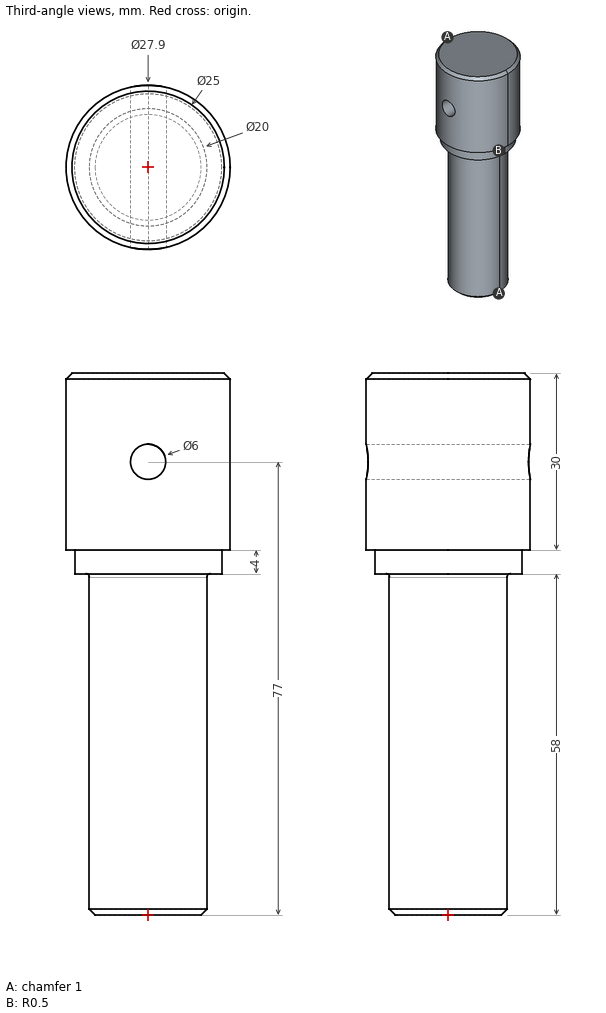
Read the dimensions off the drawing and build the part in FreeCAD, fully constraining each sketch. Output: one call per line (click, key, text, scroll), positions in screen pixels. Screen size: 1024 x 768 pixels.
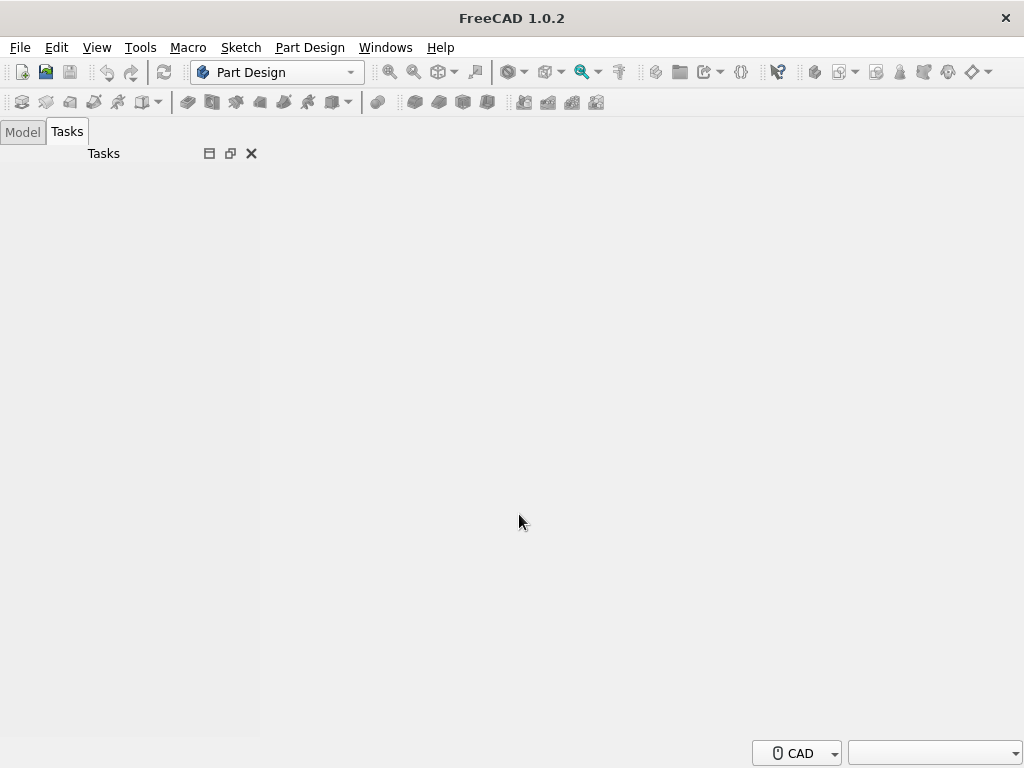
click(22, 72)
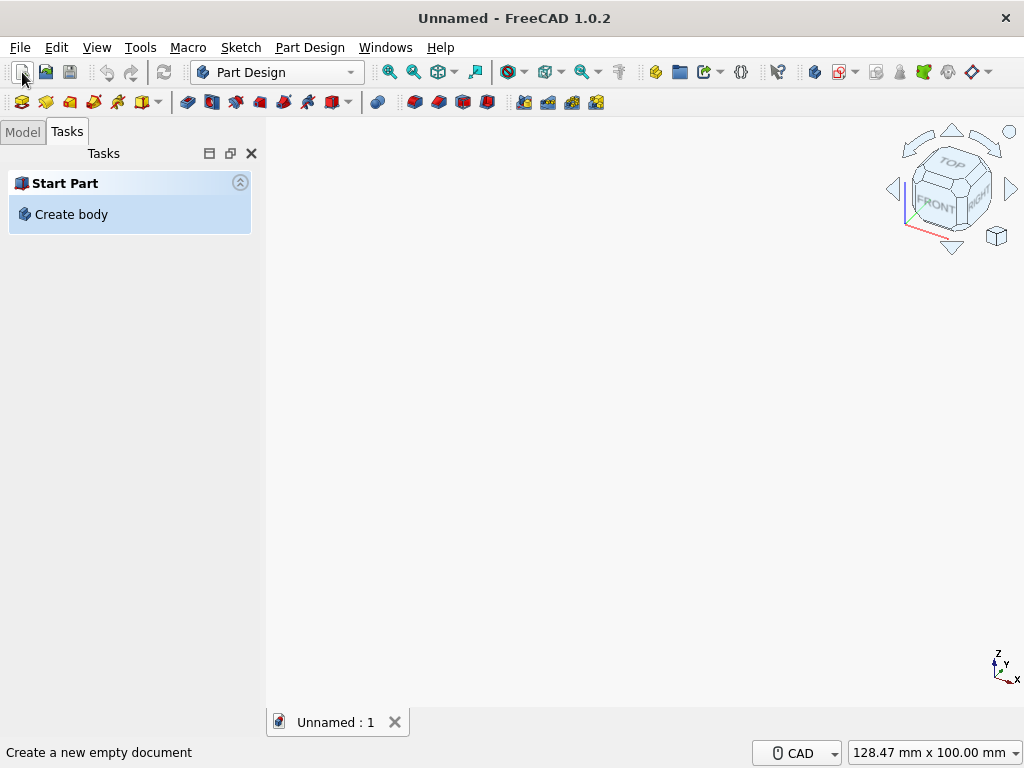
click(840, 72)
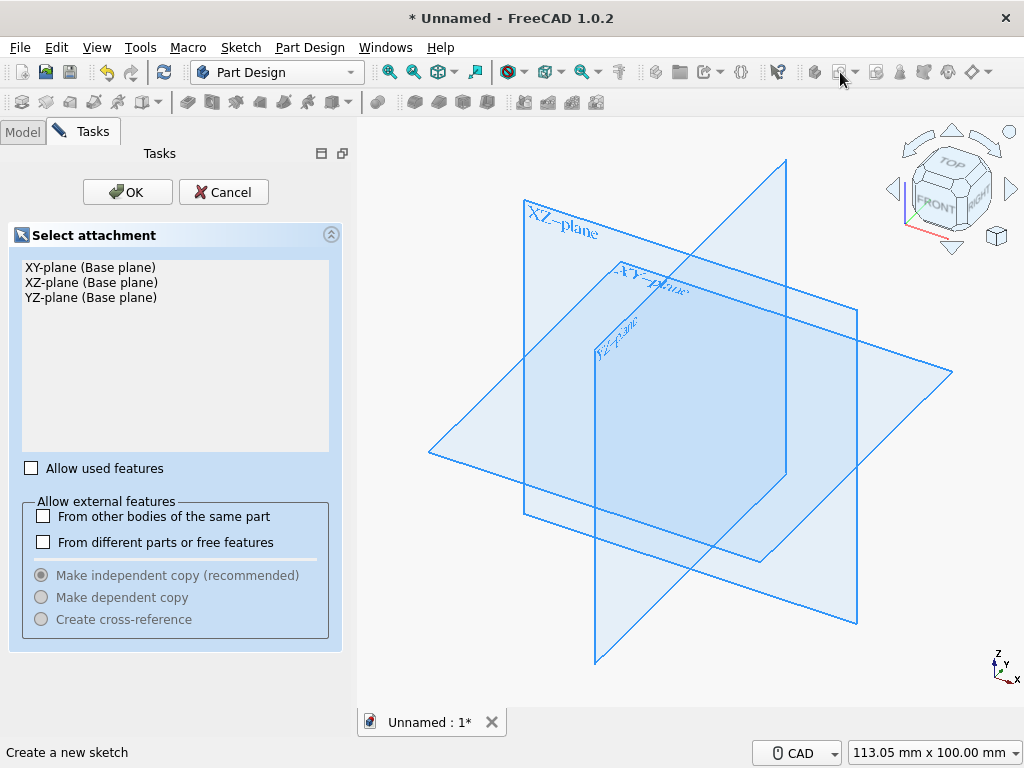
click(82, 268)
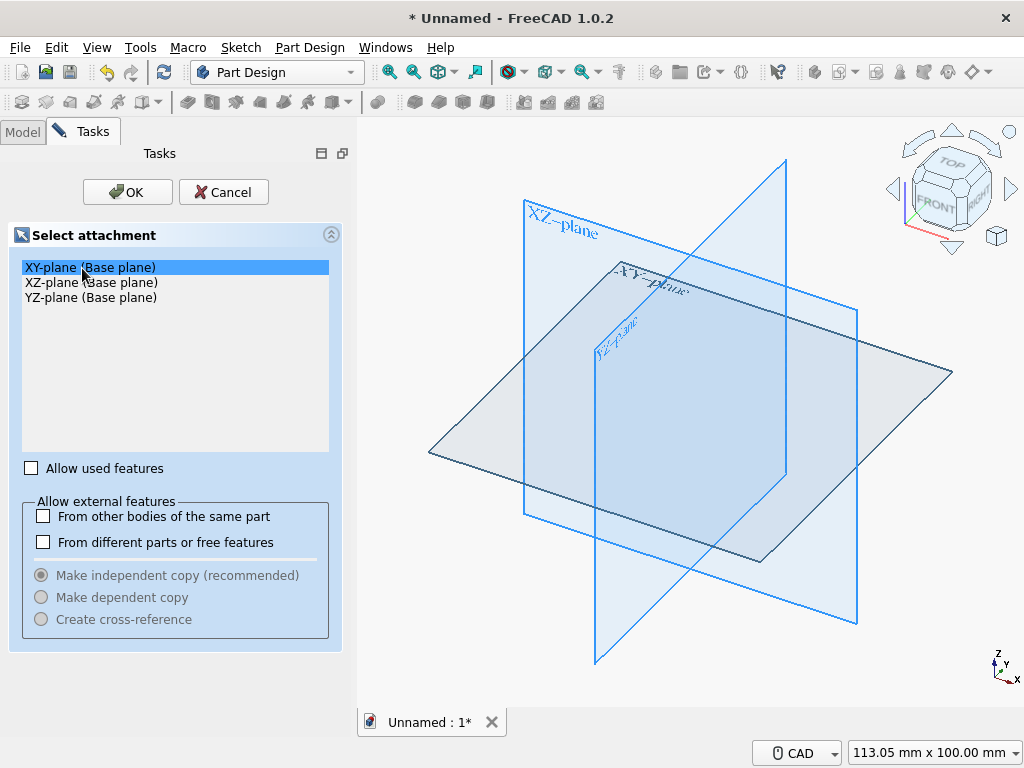
click(128, 192)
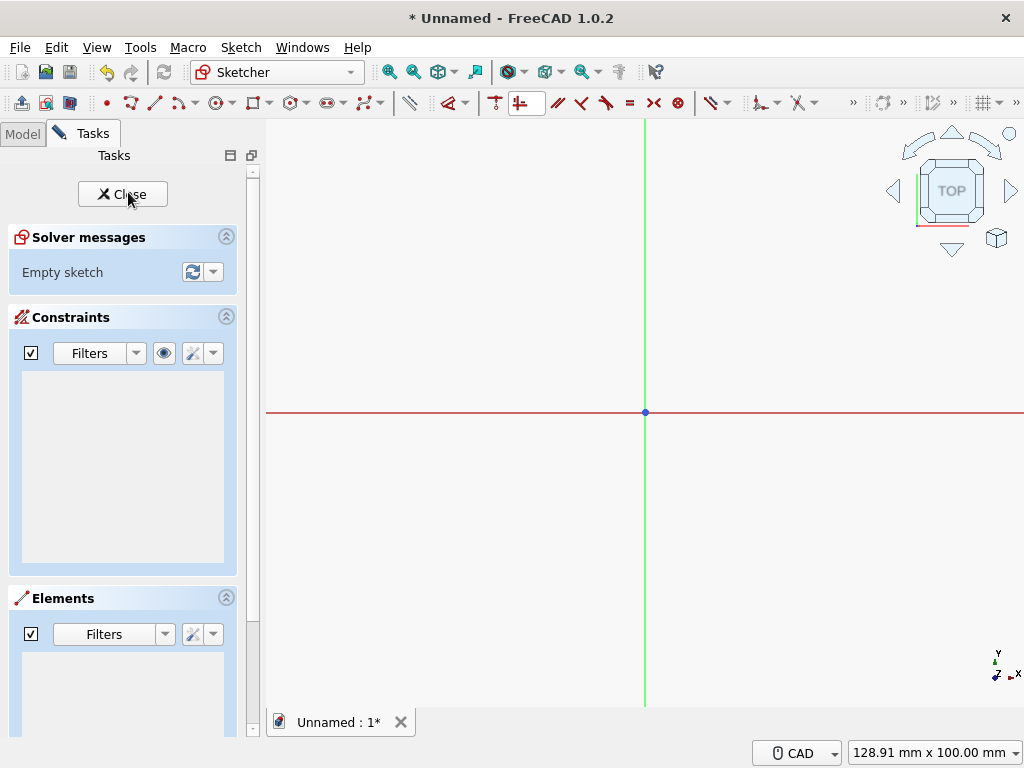
scroll(675, 413, up, 6)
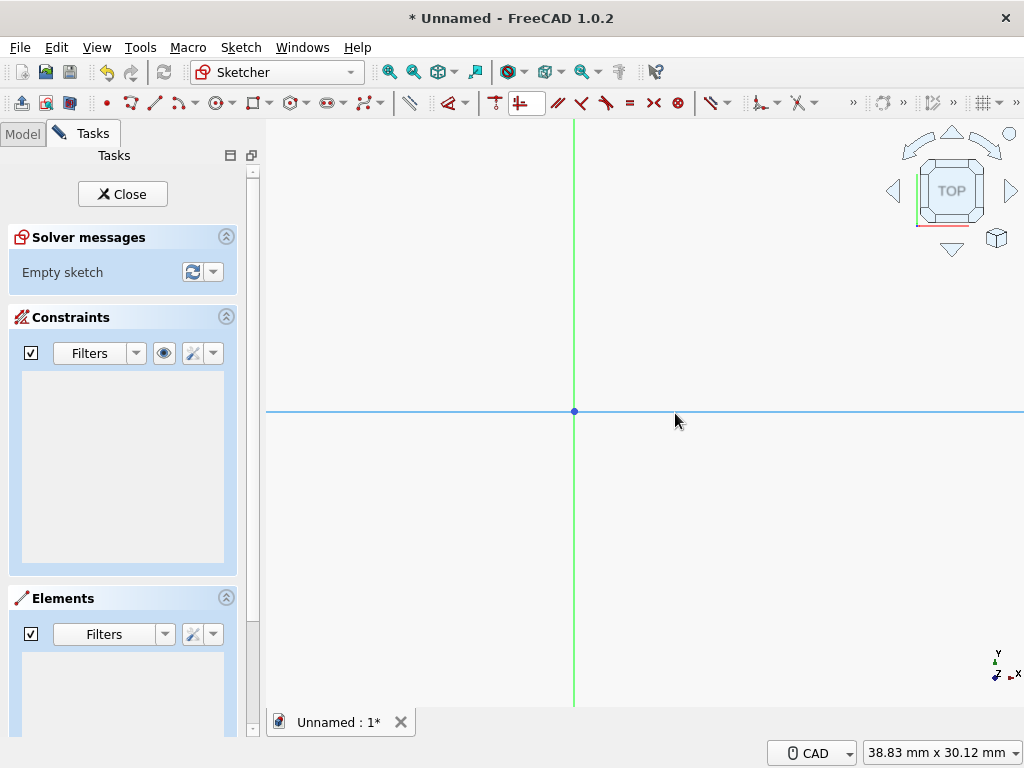
click(216, 104)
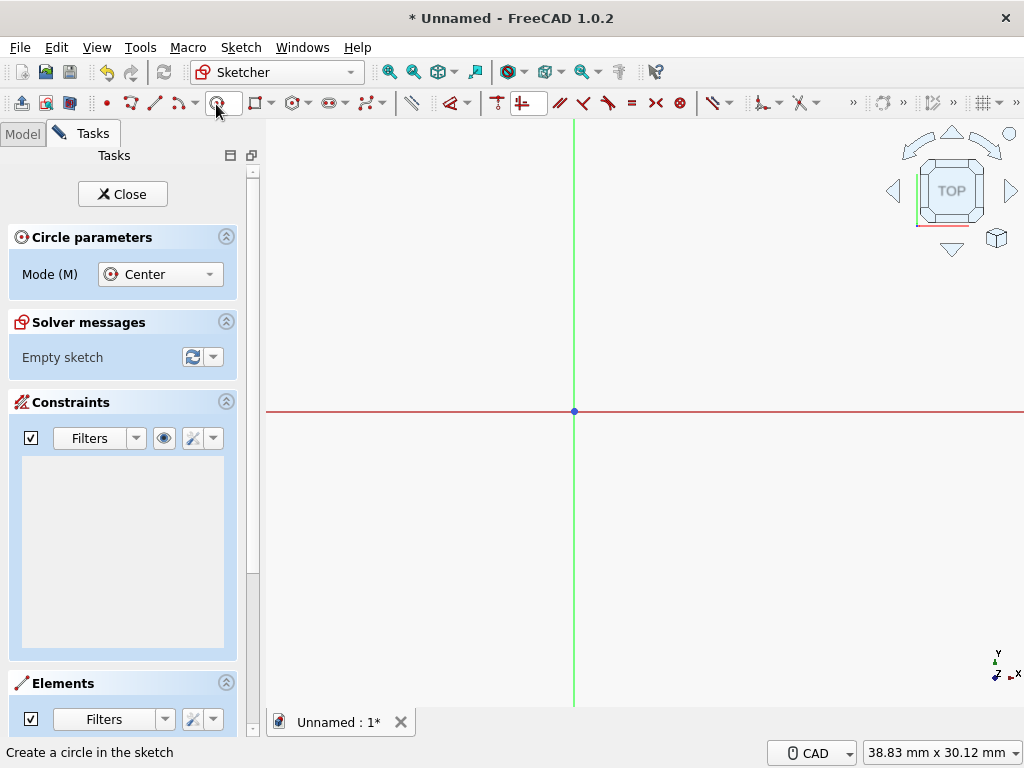
click(574, 412)
click(712, 274)
key(Escape)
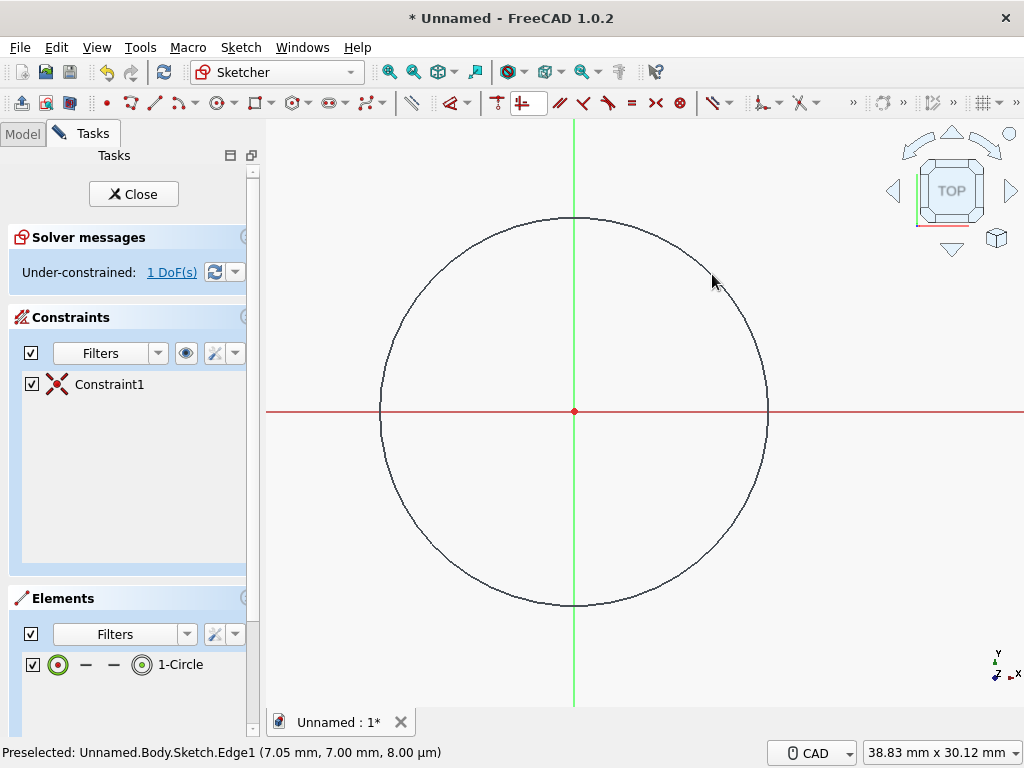
click(450, 104)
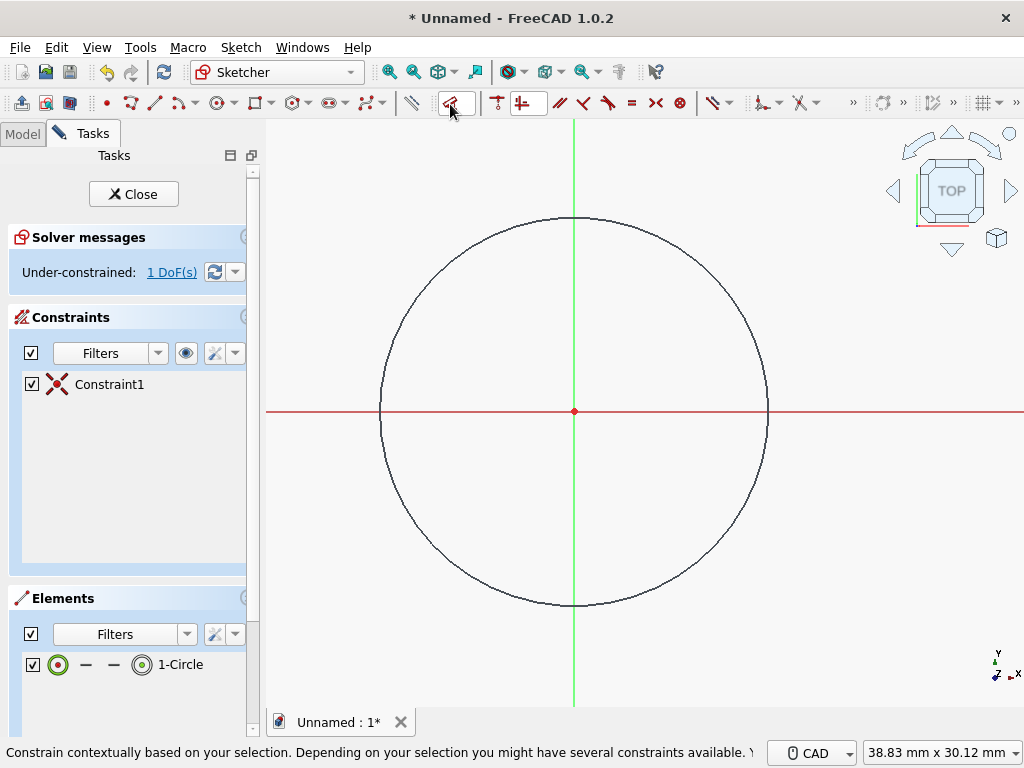
click(711, 274)
click(734, 251)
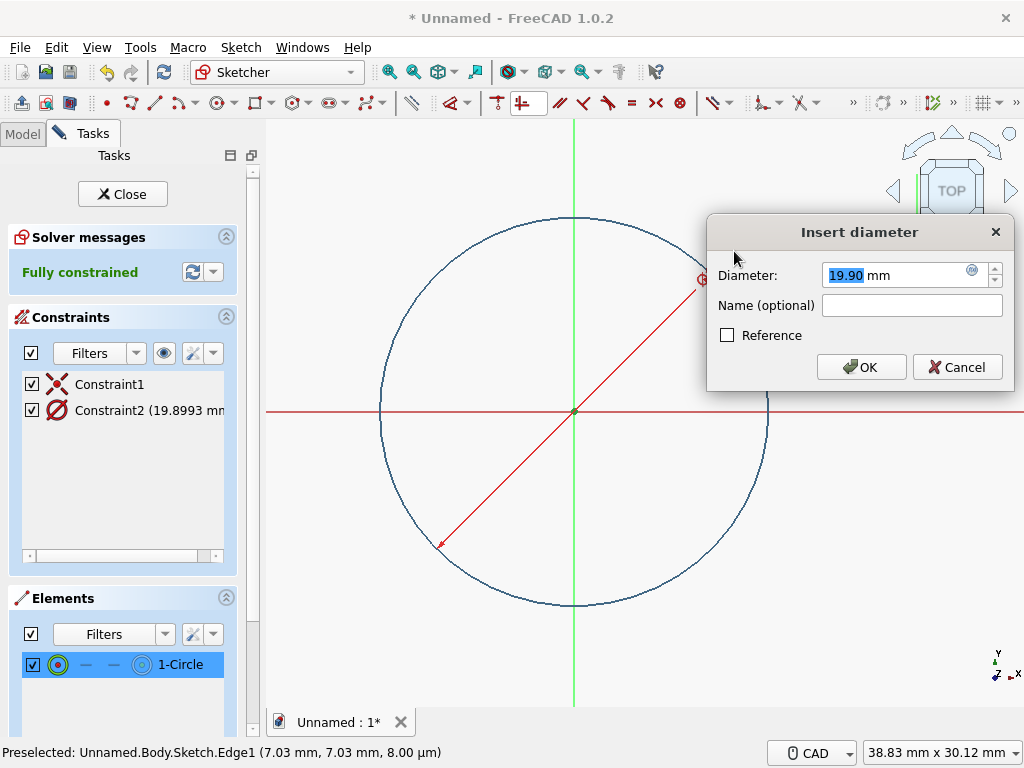
text(20)
key(Return)
key(Escape)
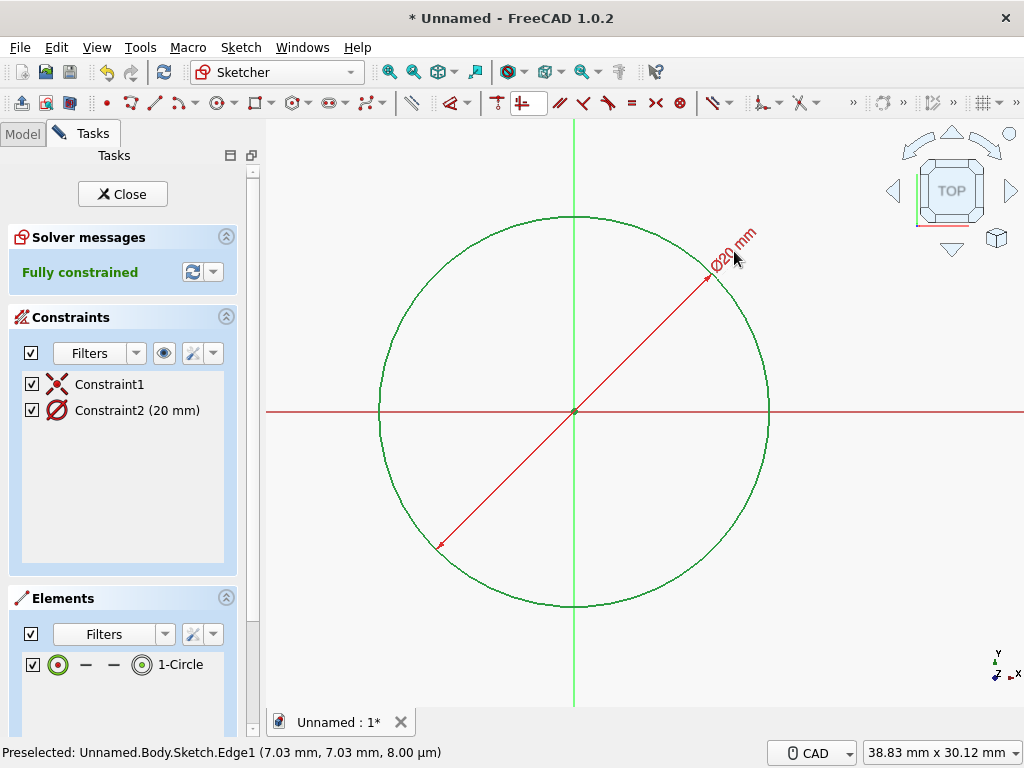
click(123, 194)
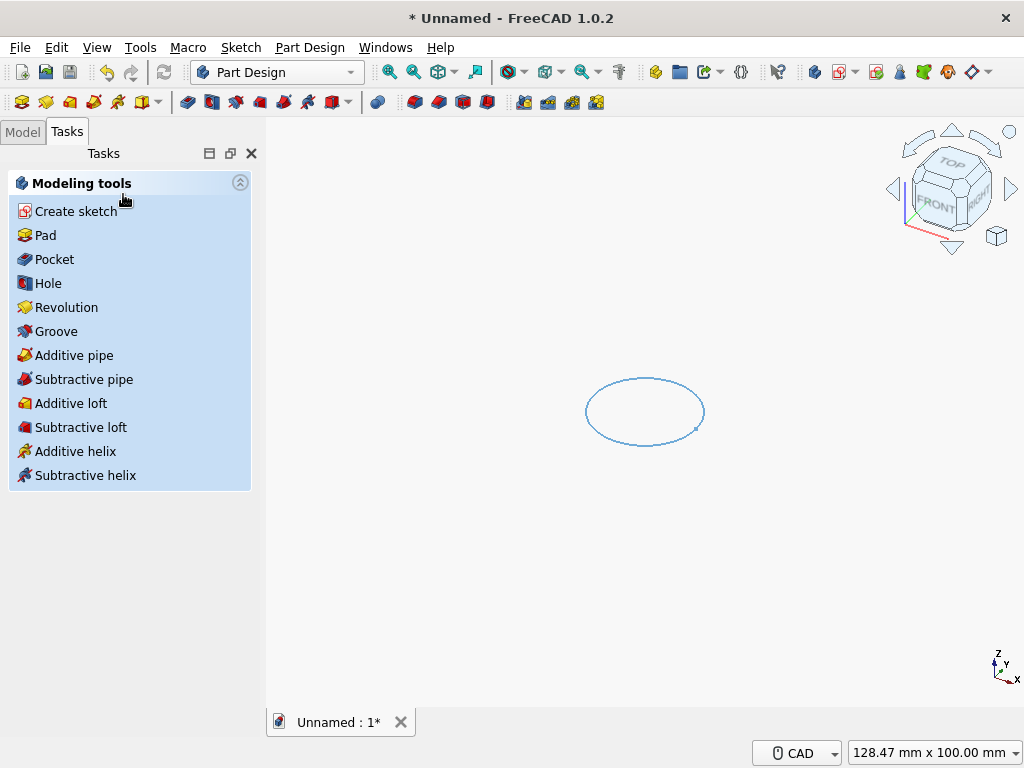
click(22, 102)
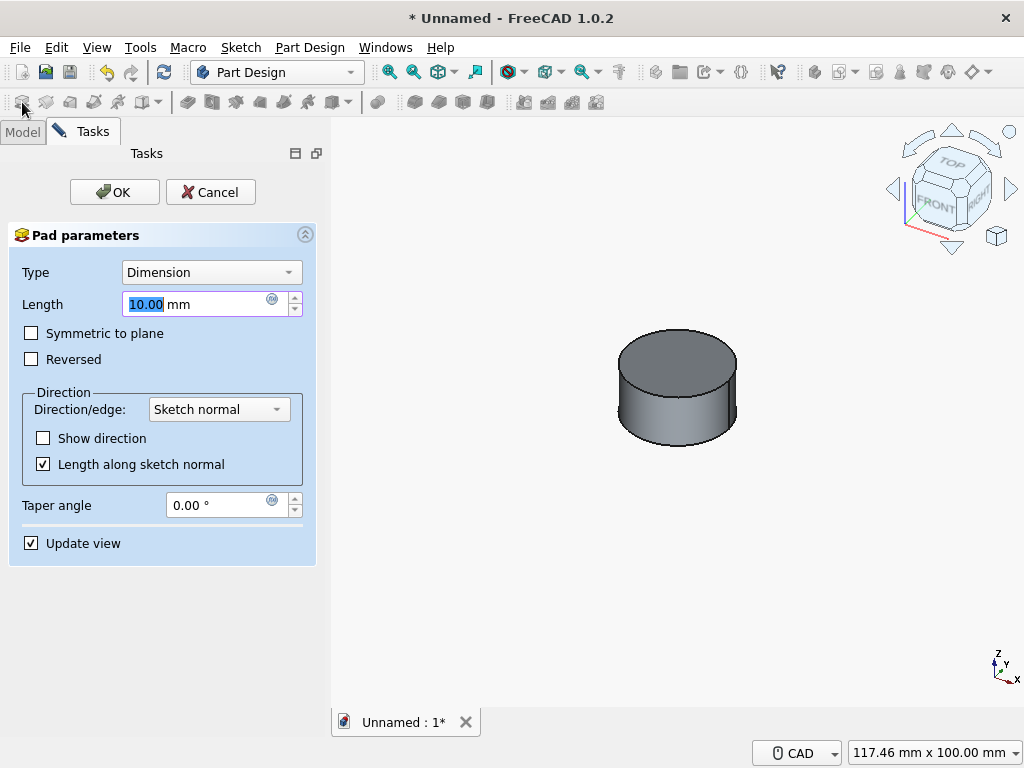
text(58)
key(Tab)